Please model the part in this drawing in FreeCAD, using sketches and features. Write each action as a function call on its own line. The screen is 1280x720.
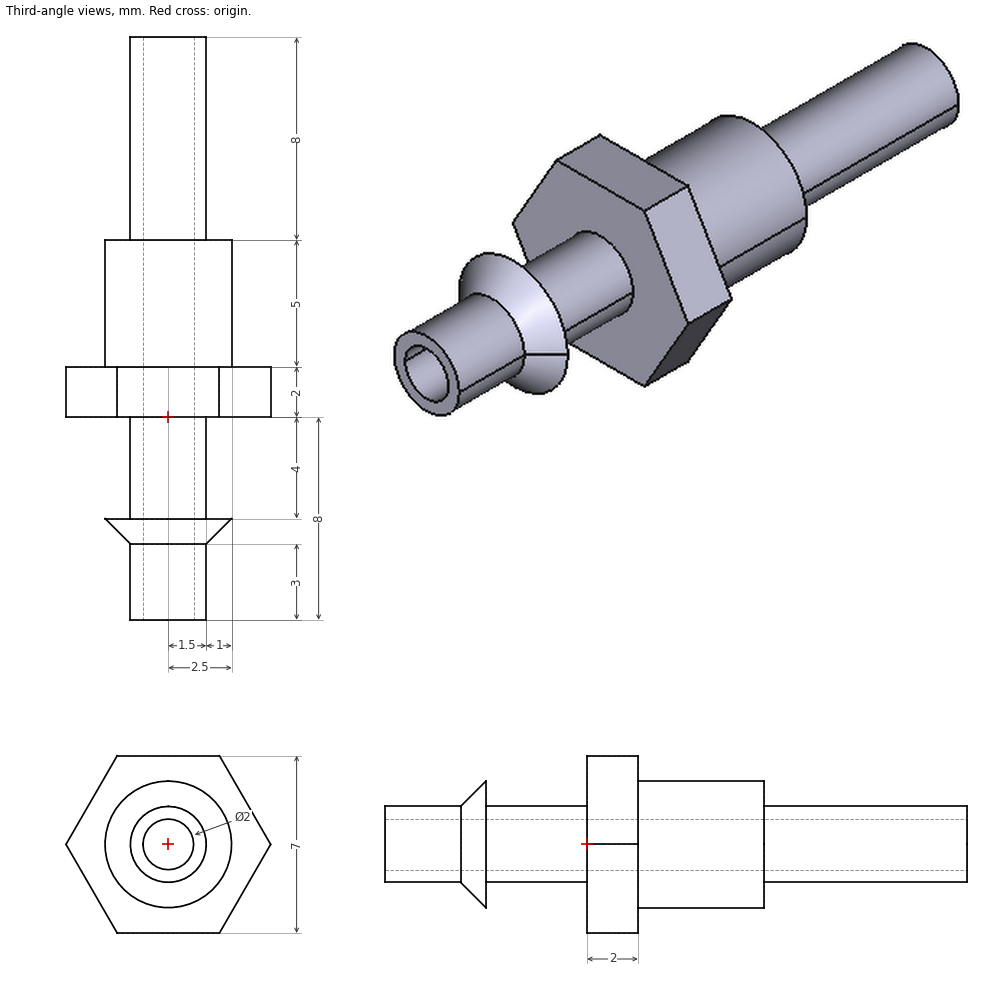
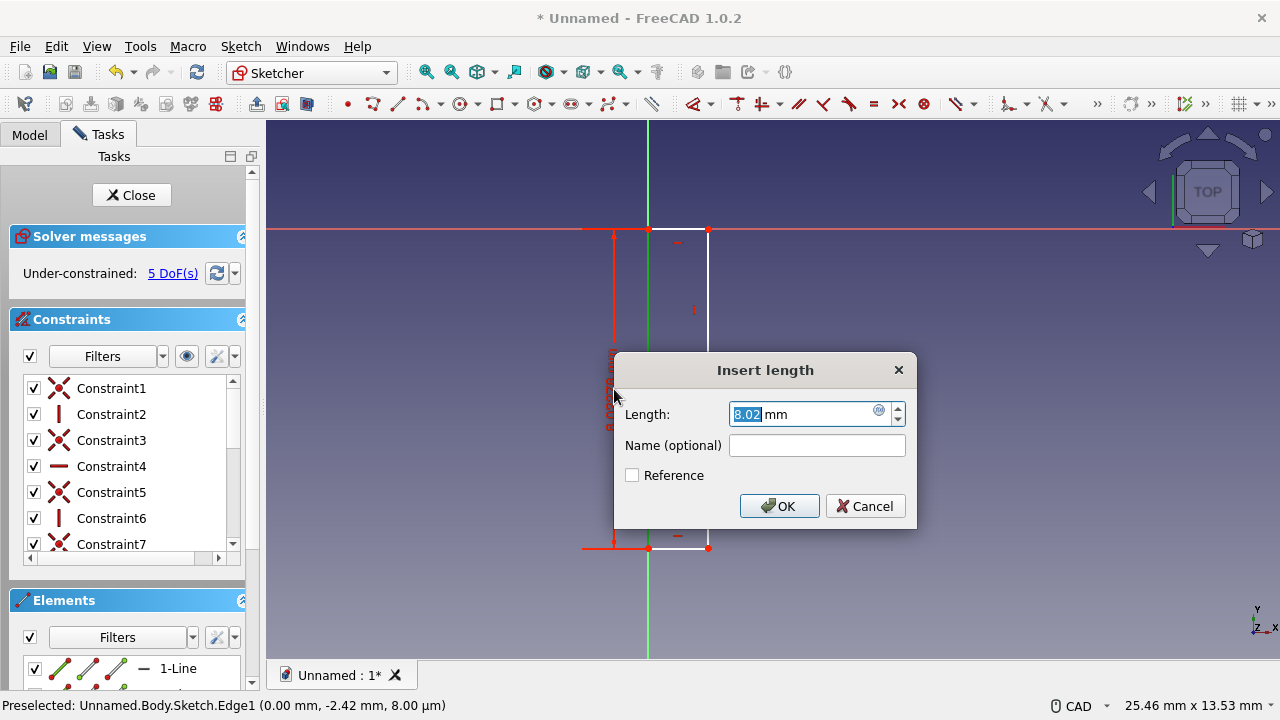
text(8)
key(Return)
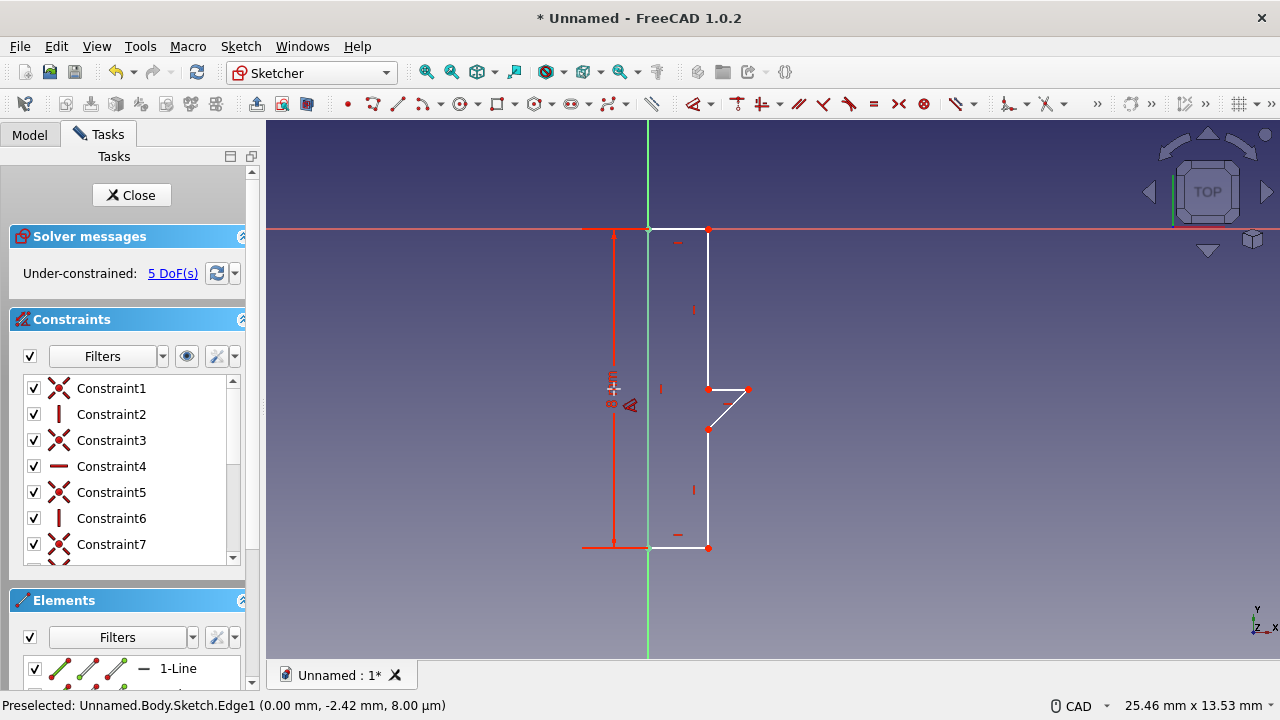
click(708, 513)
click(742, 489)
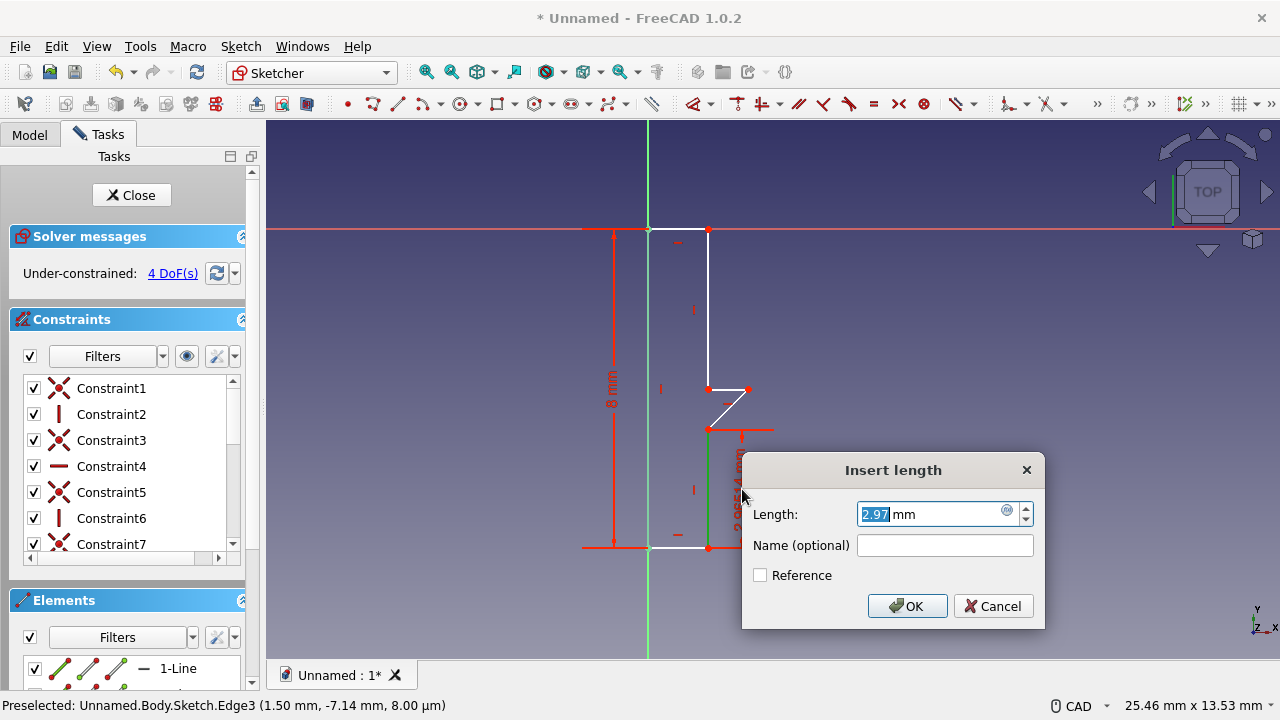
text(3)
key(Return)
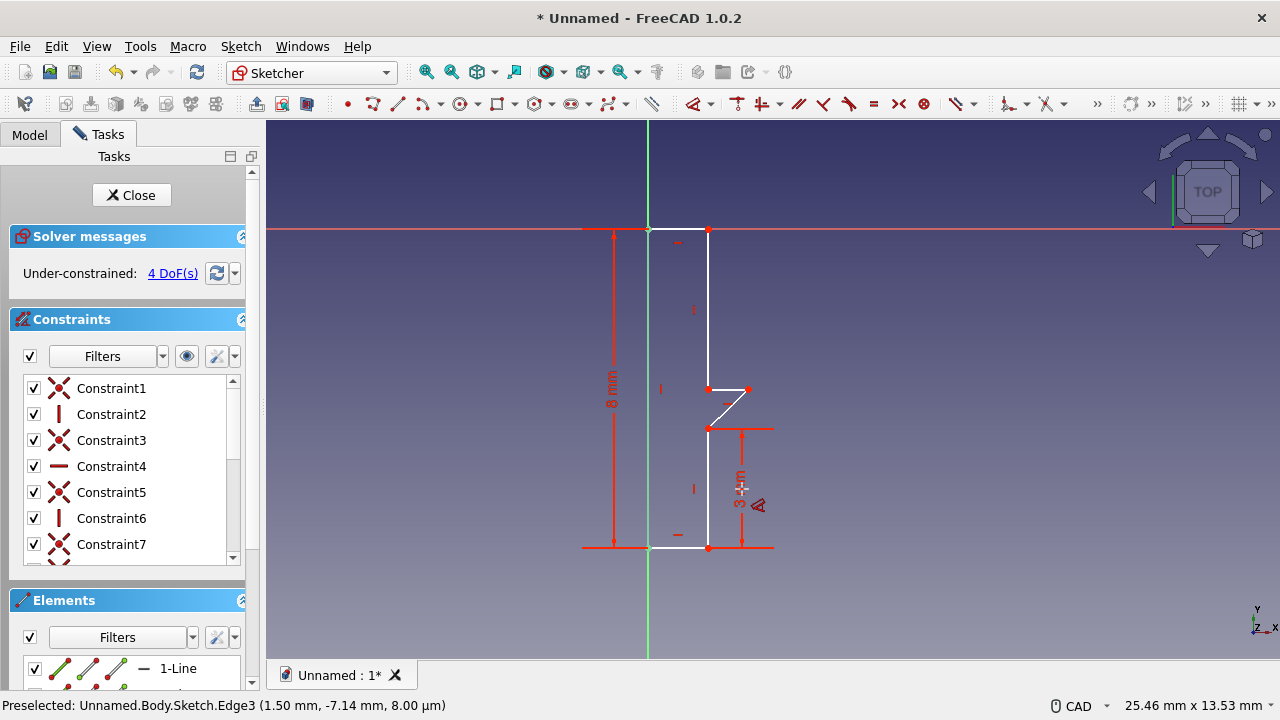
click(720, 390)
click(737, 424)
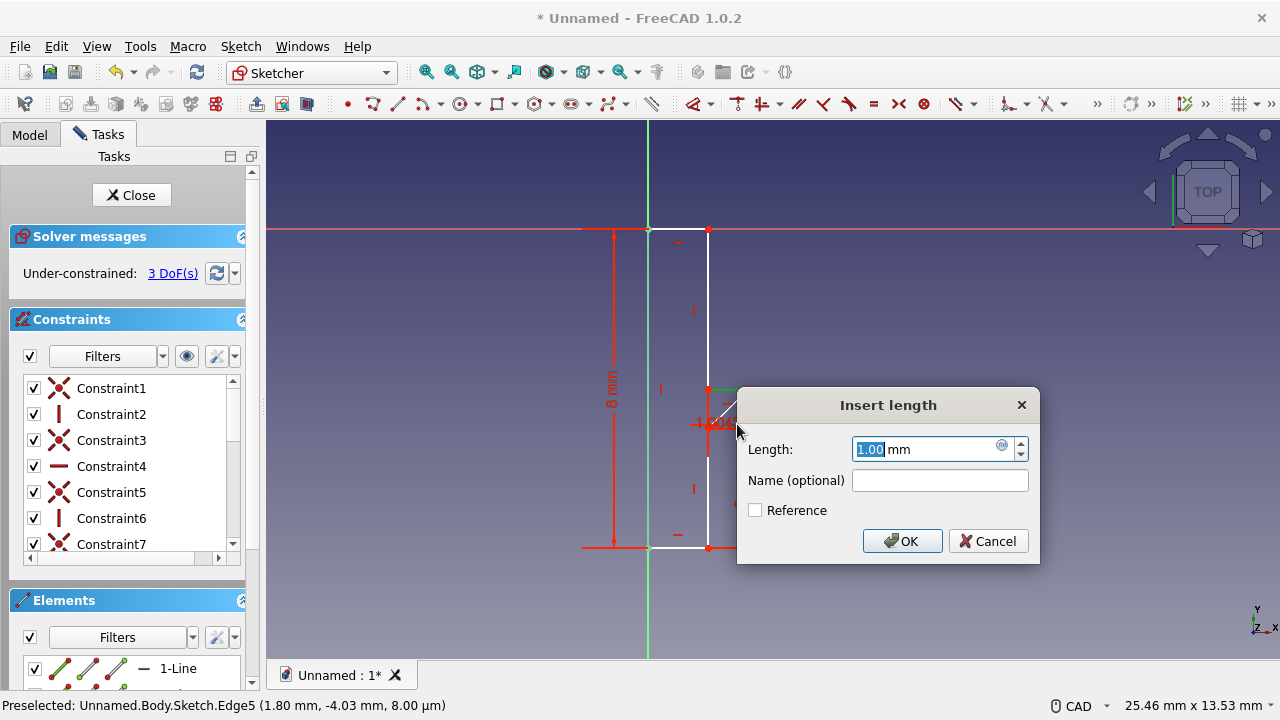
text(1)
key(Return)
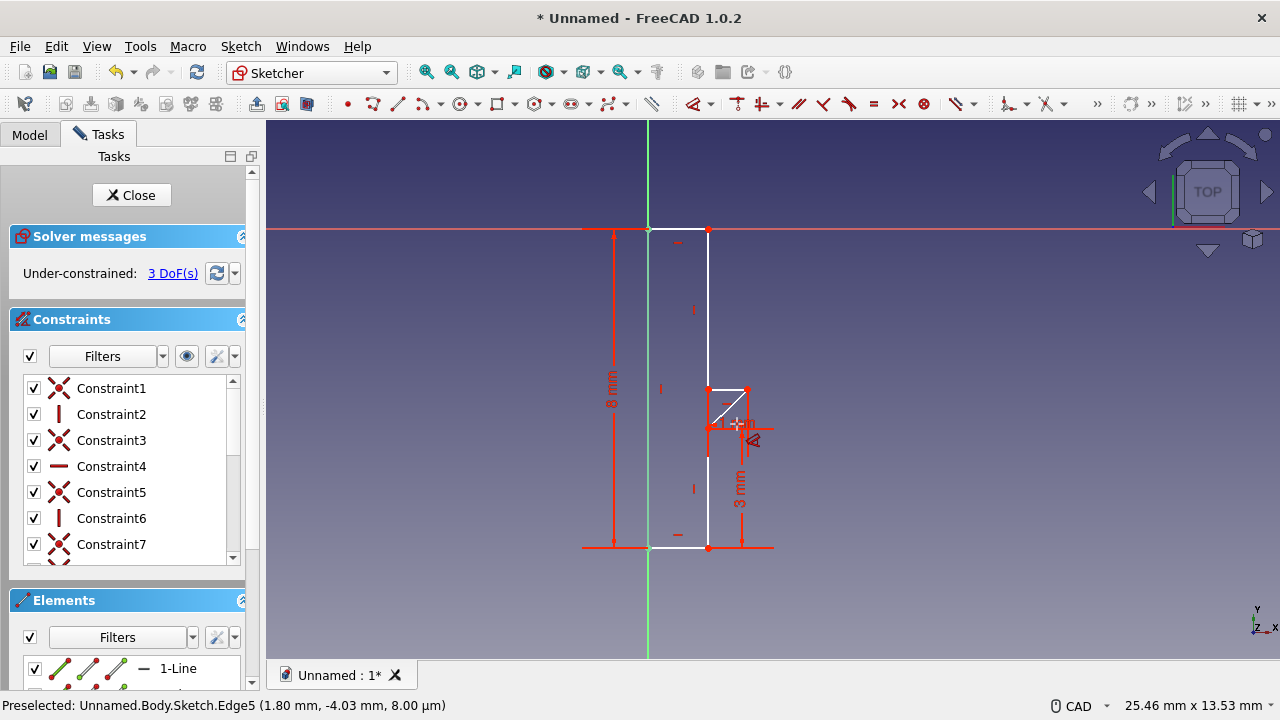
click(708, 342)
click(742, 310)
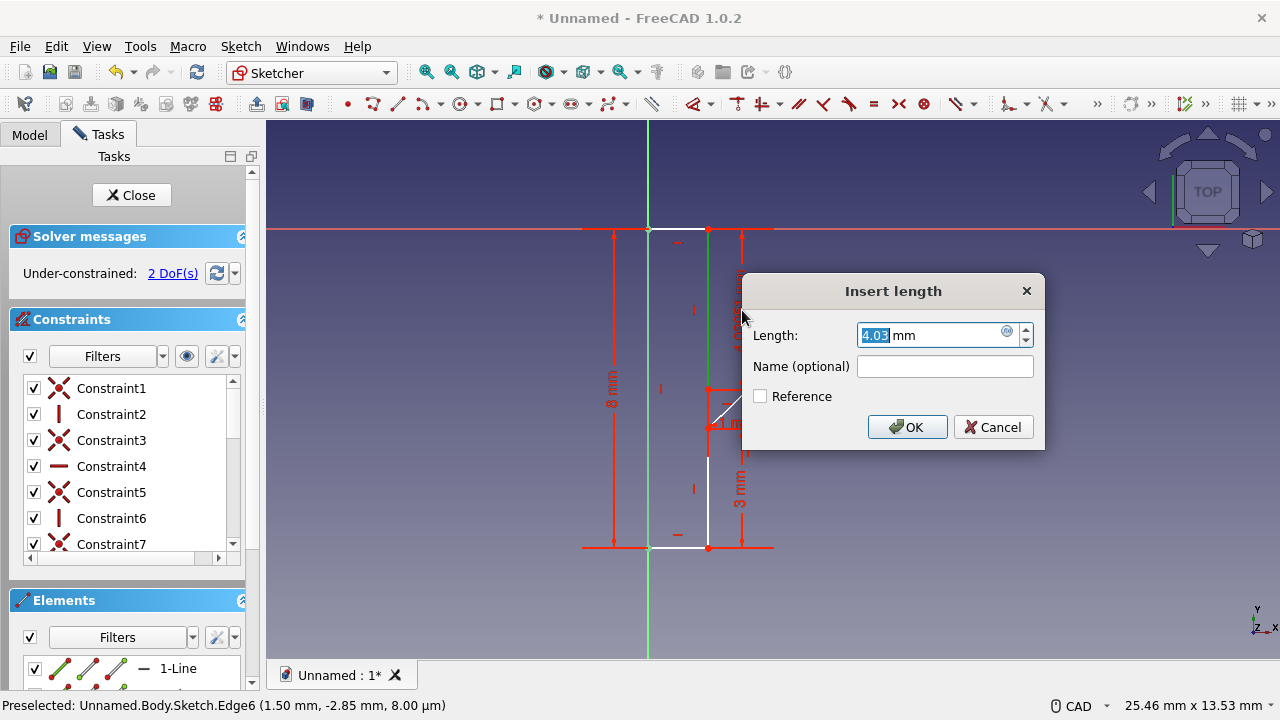
text(4)
key(Return)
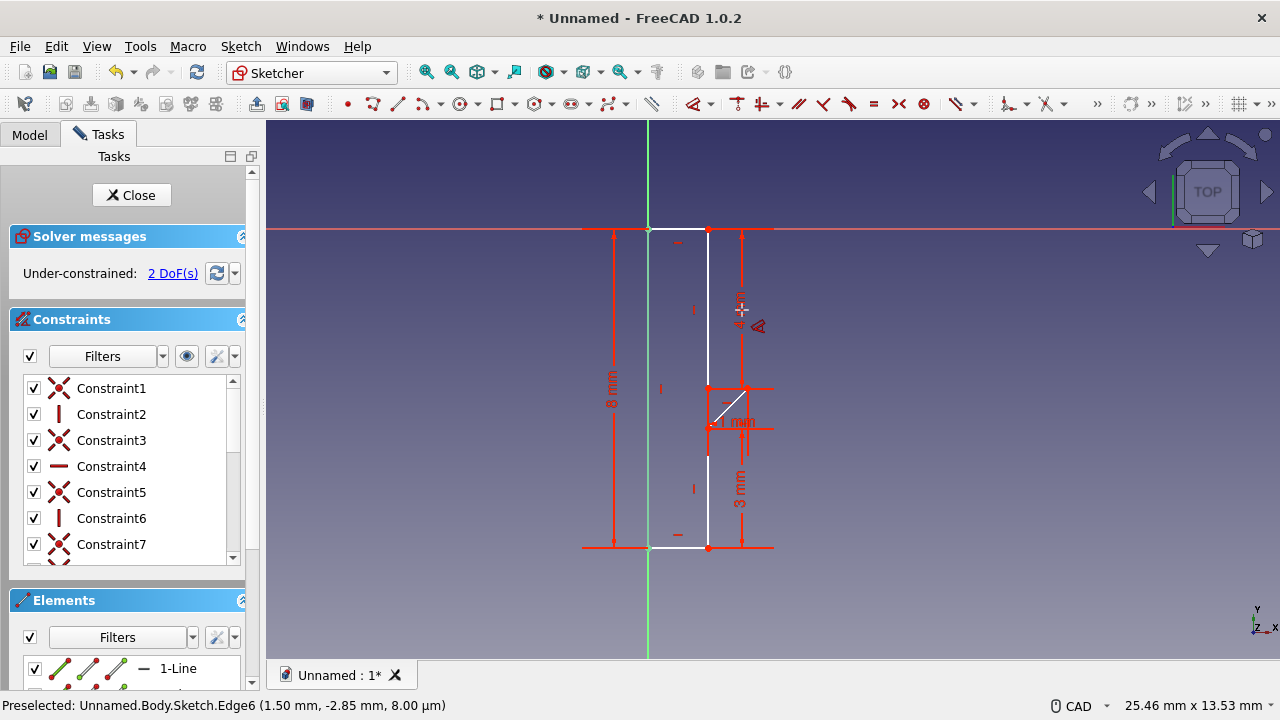
click(720, 417)
click(728, 463)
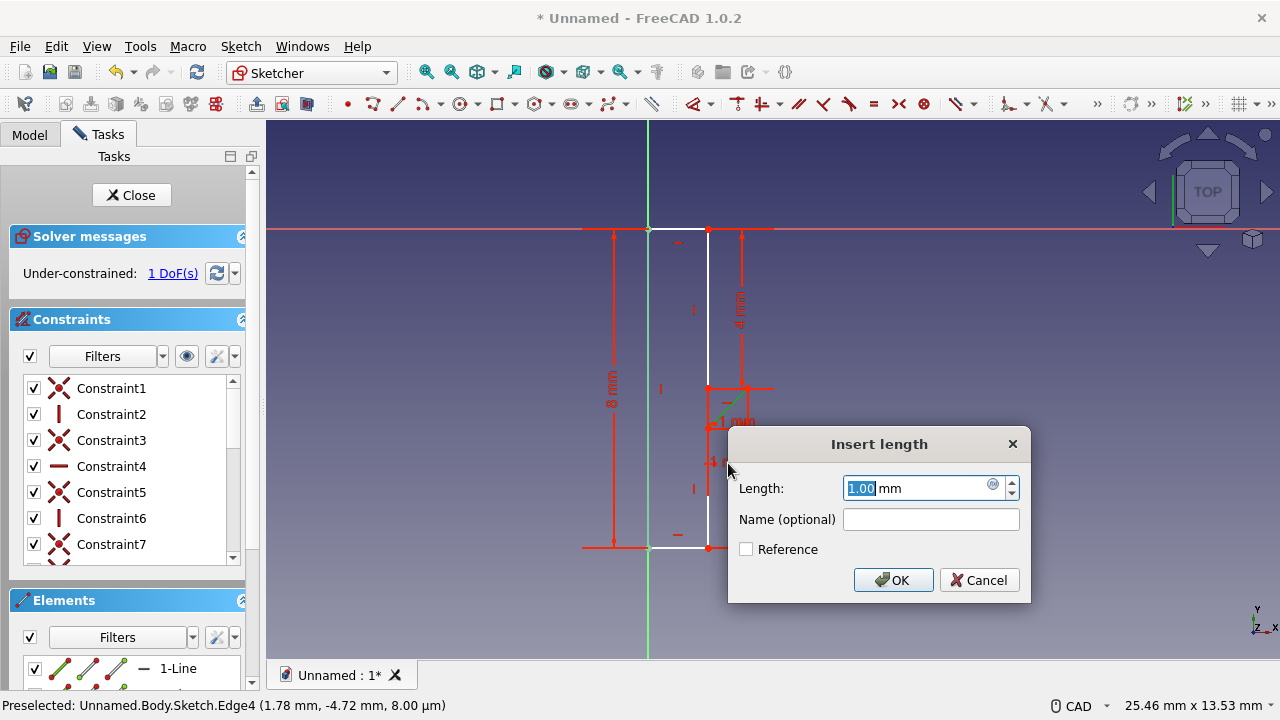
text(1)
key(Return)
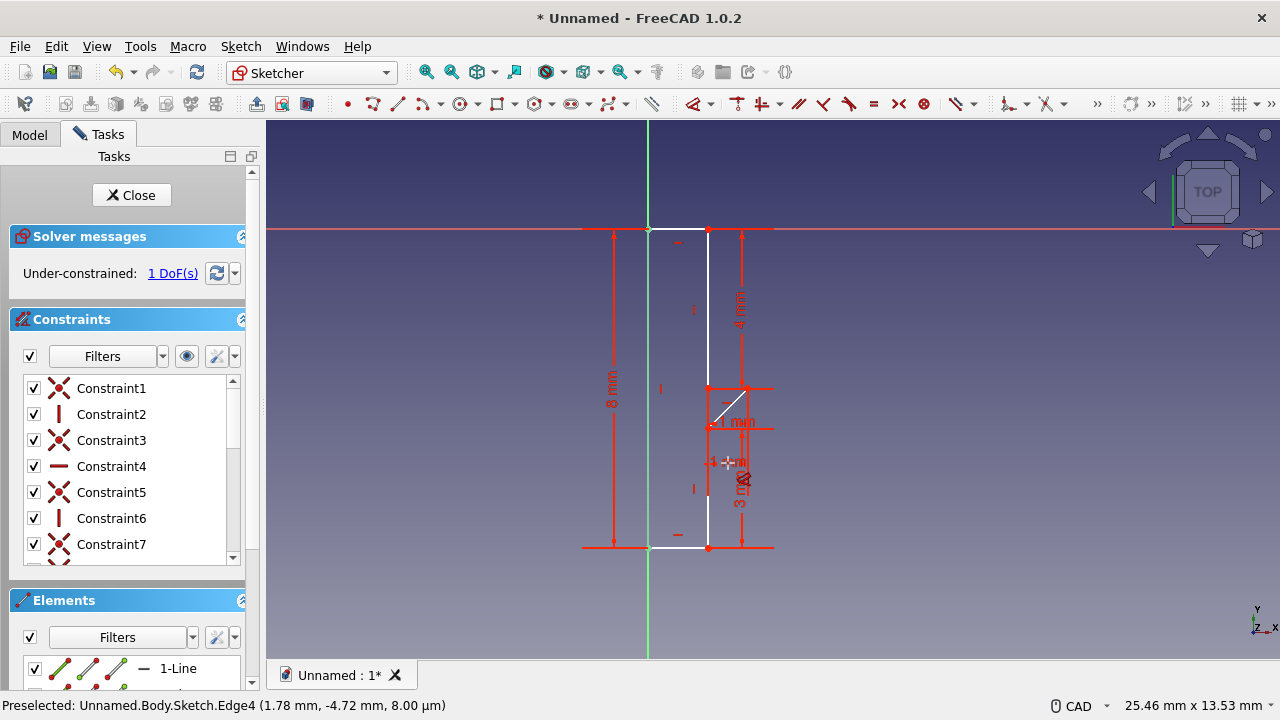
click(666, 548)
click(678, 582)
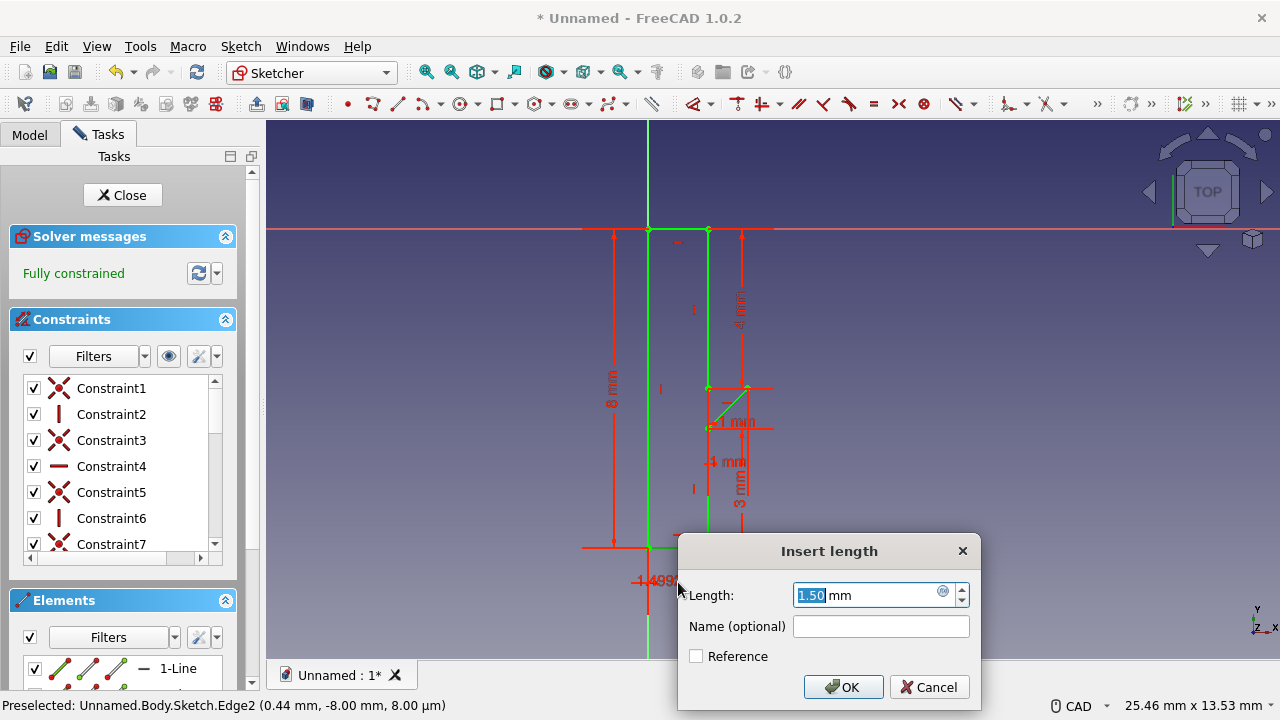
text(1.5)
key(Return)
key(Escape)